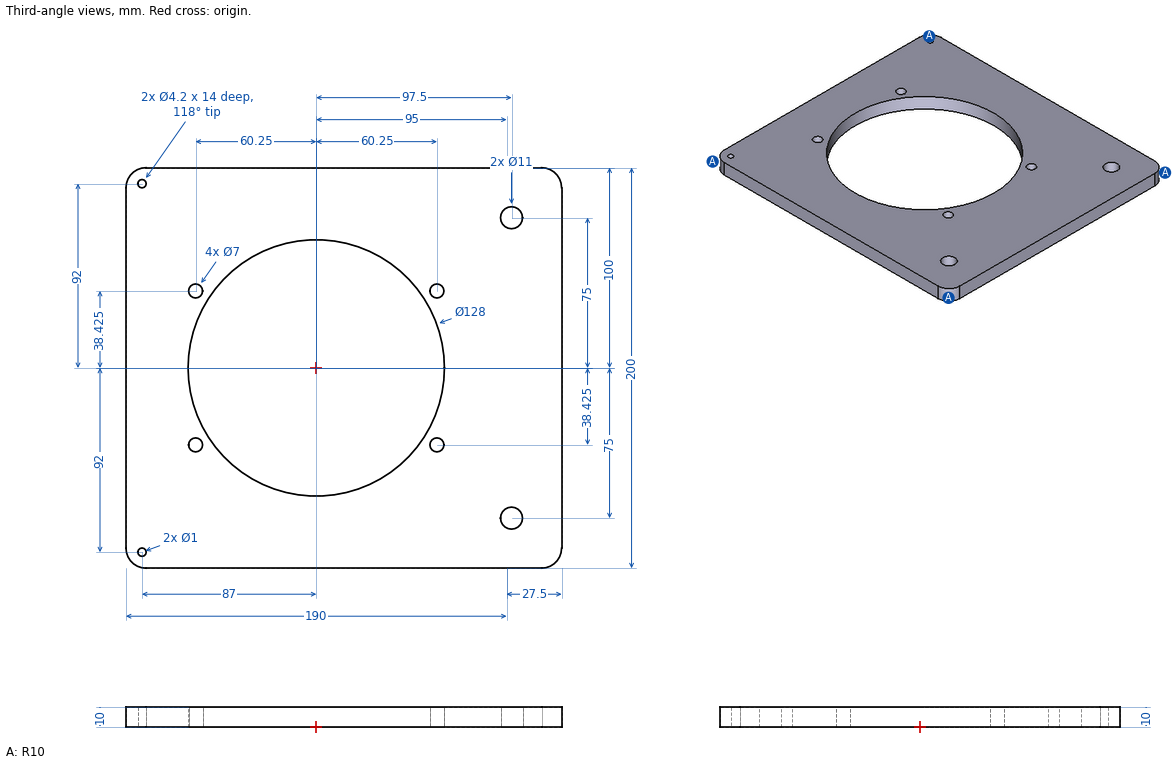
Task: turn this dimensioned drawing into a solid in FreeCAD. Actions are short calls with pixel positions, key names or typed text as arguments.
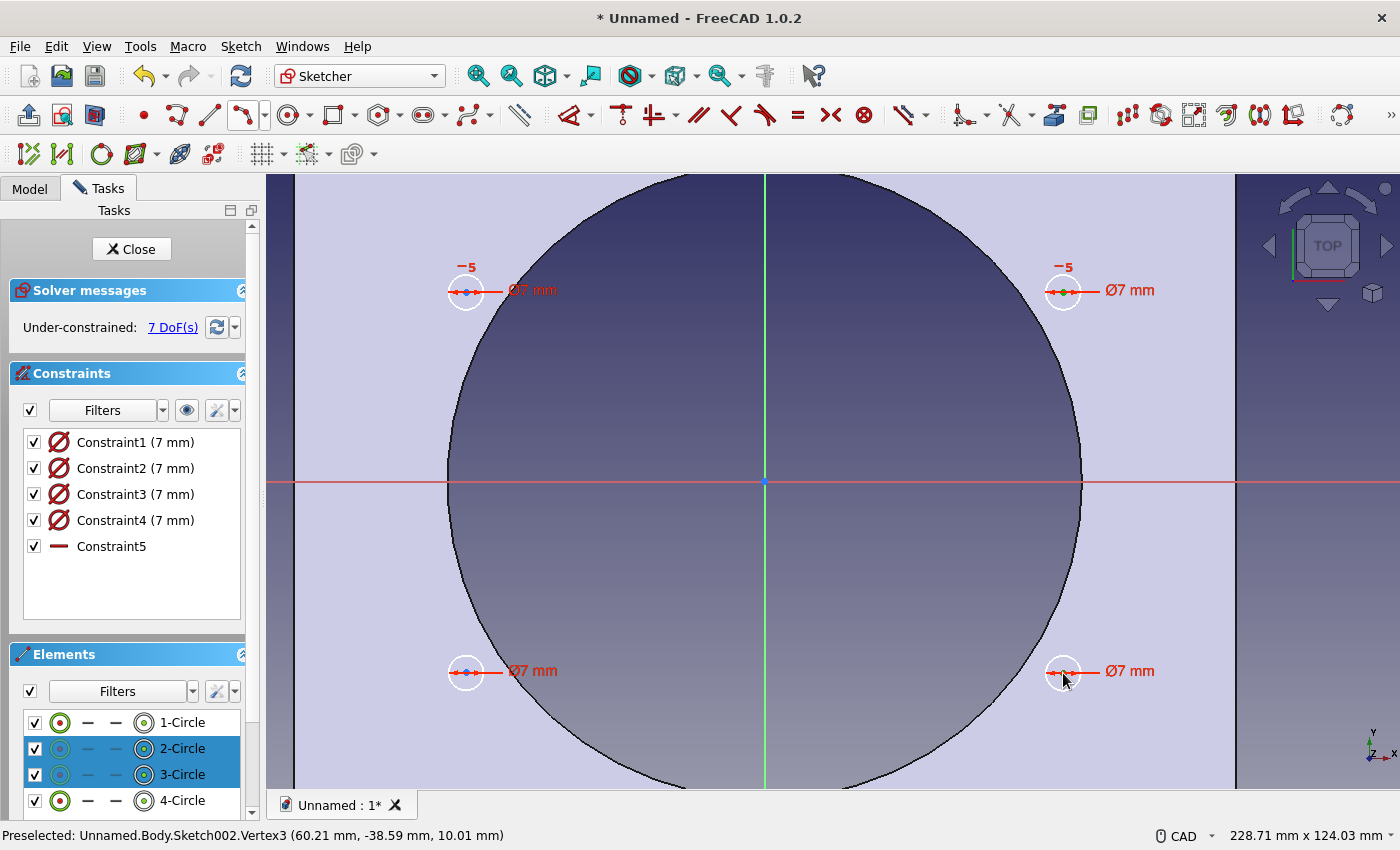
key(v)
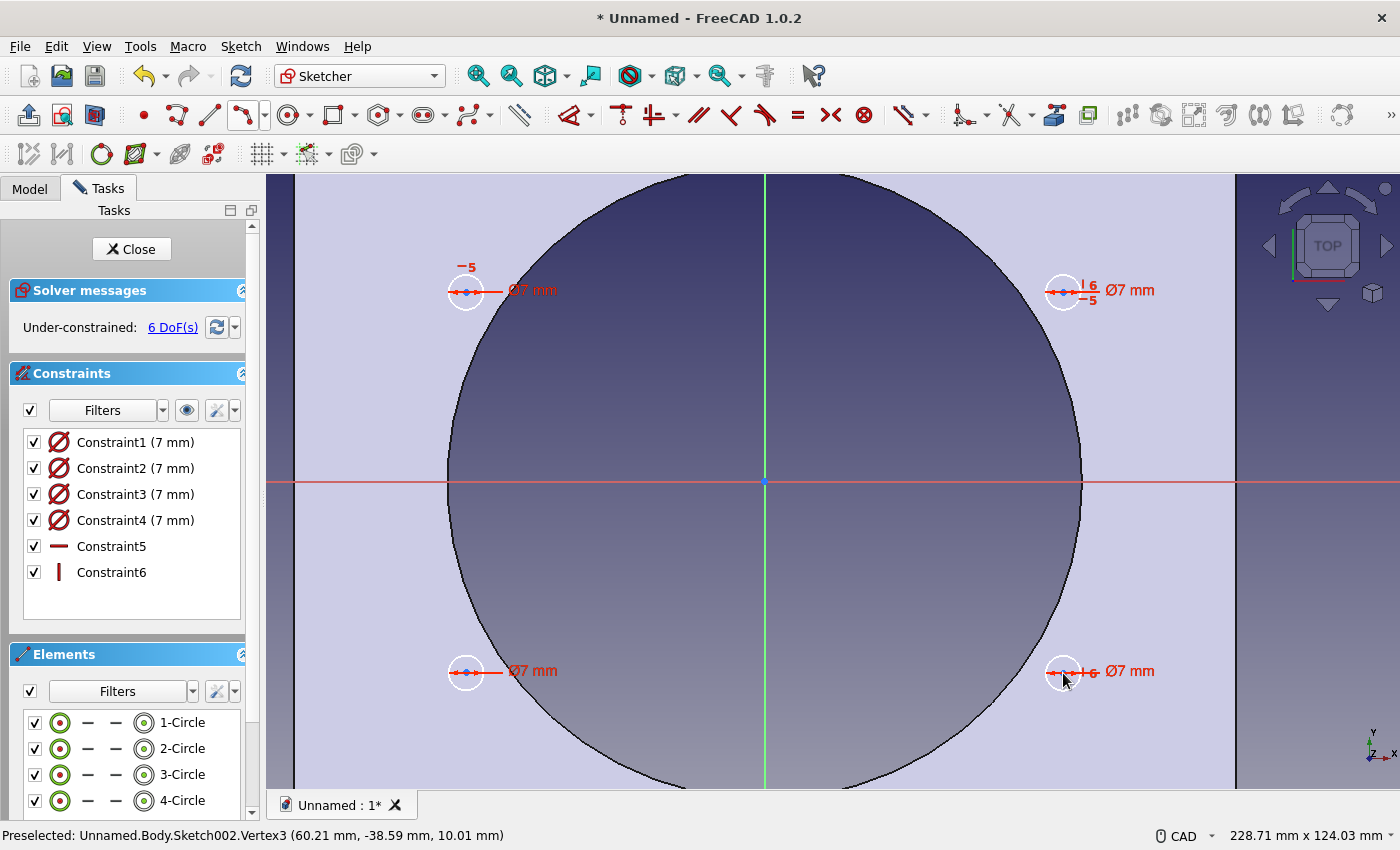
click(466, 292)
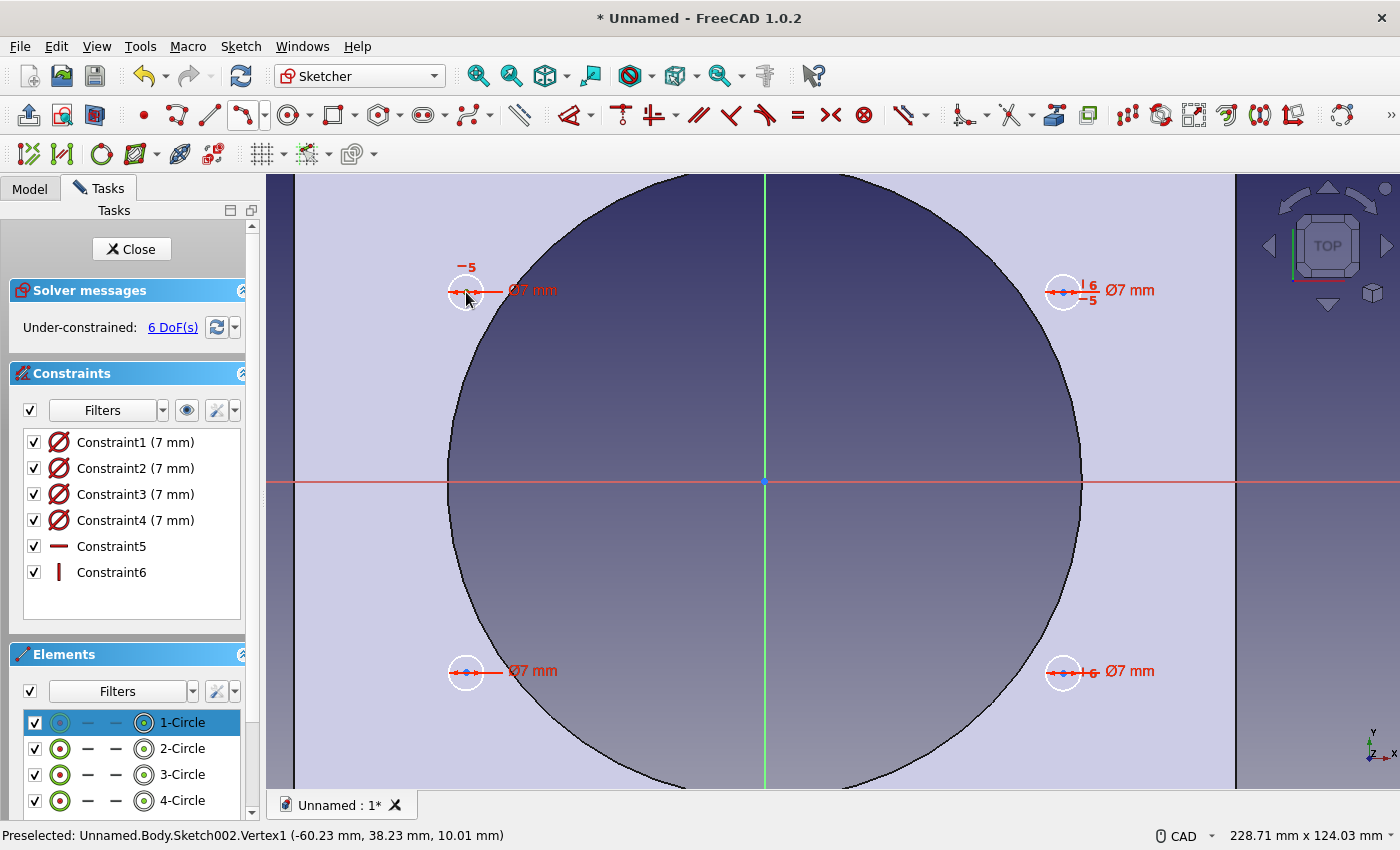
click(466, 673)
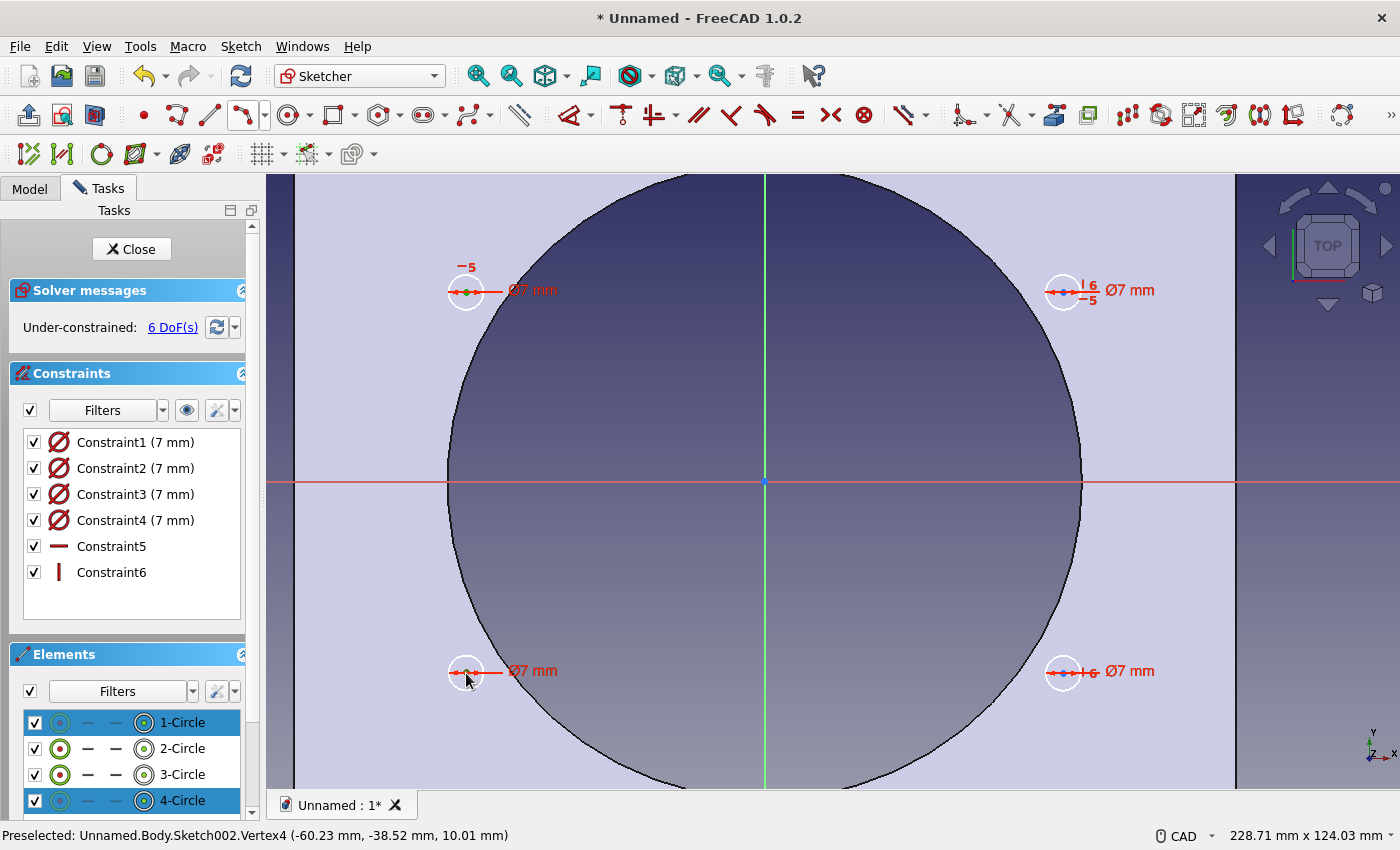
key(v)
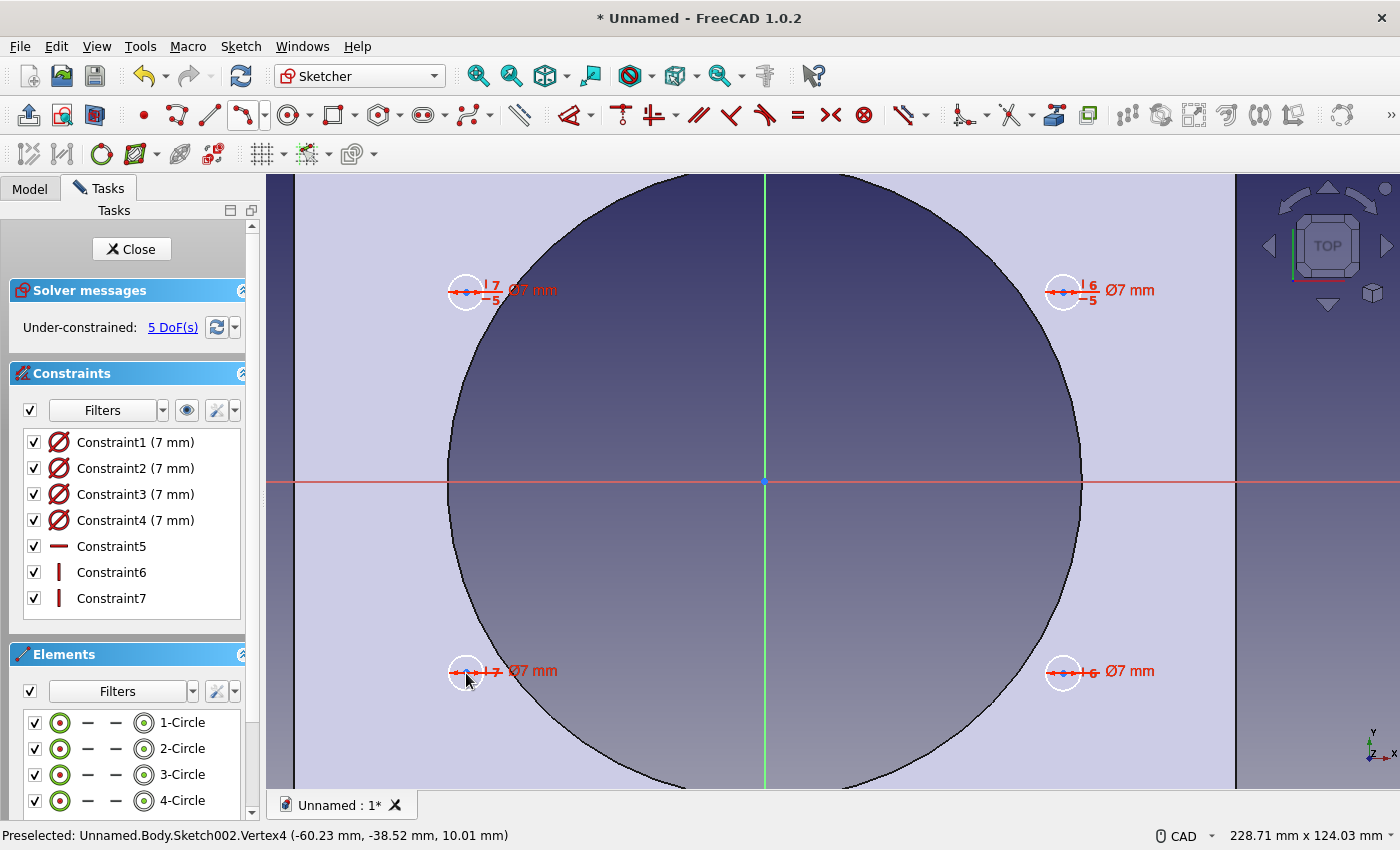
click(1063, 673)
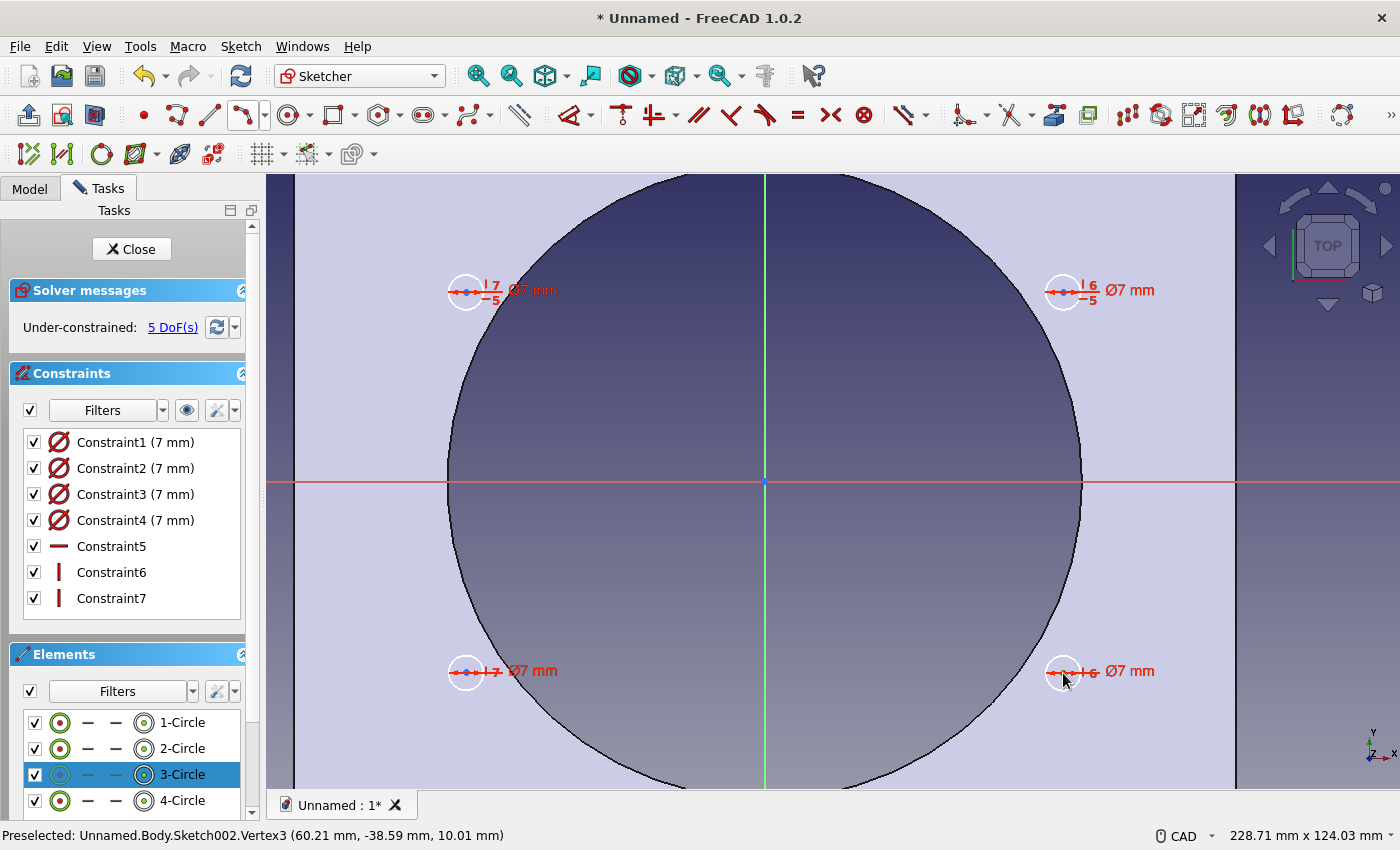
click(466, 673)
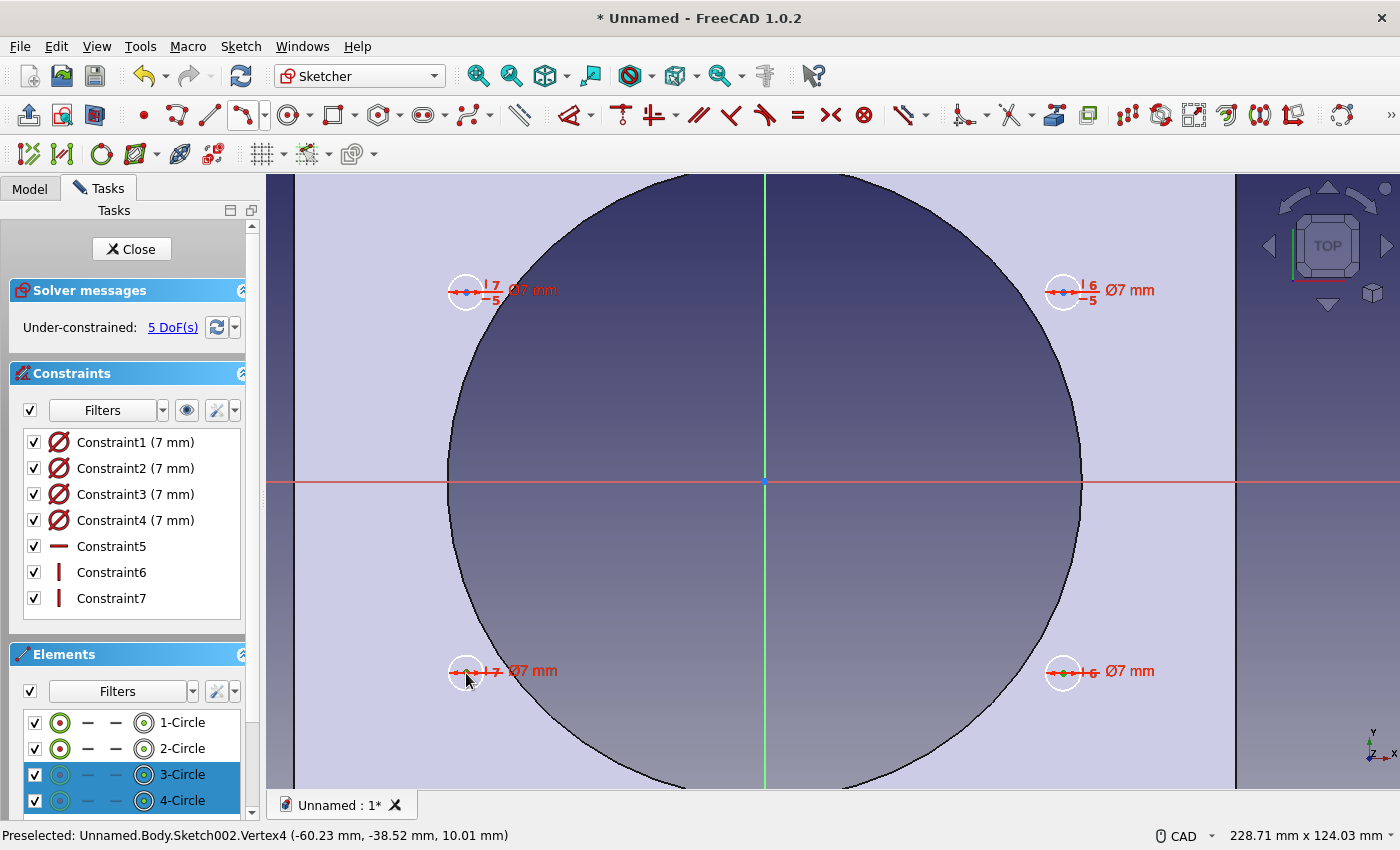
key(h)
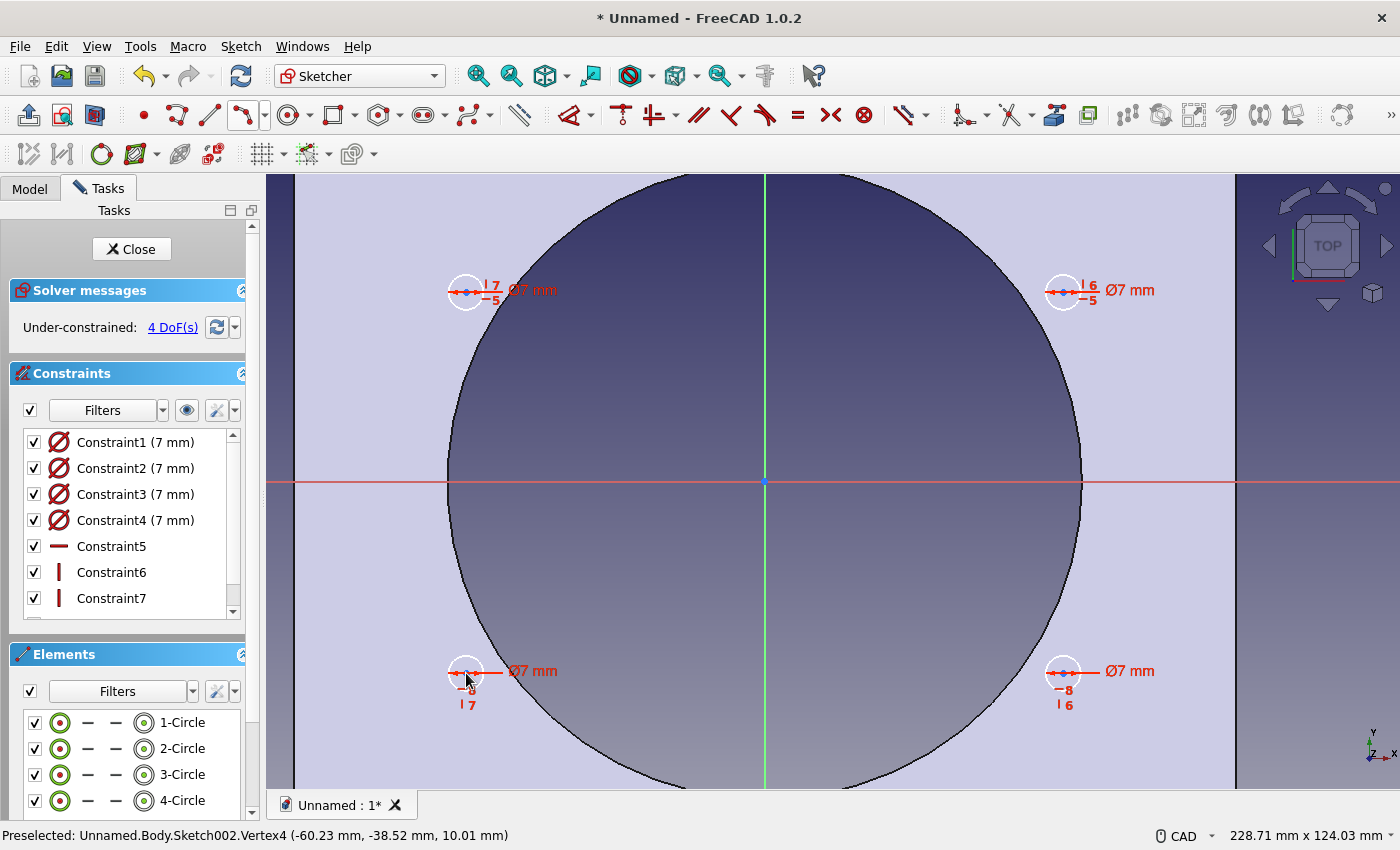
click(568, 116)